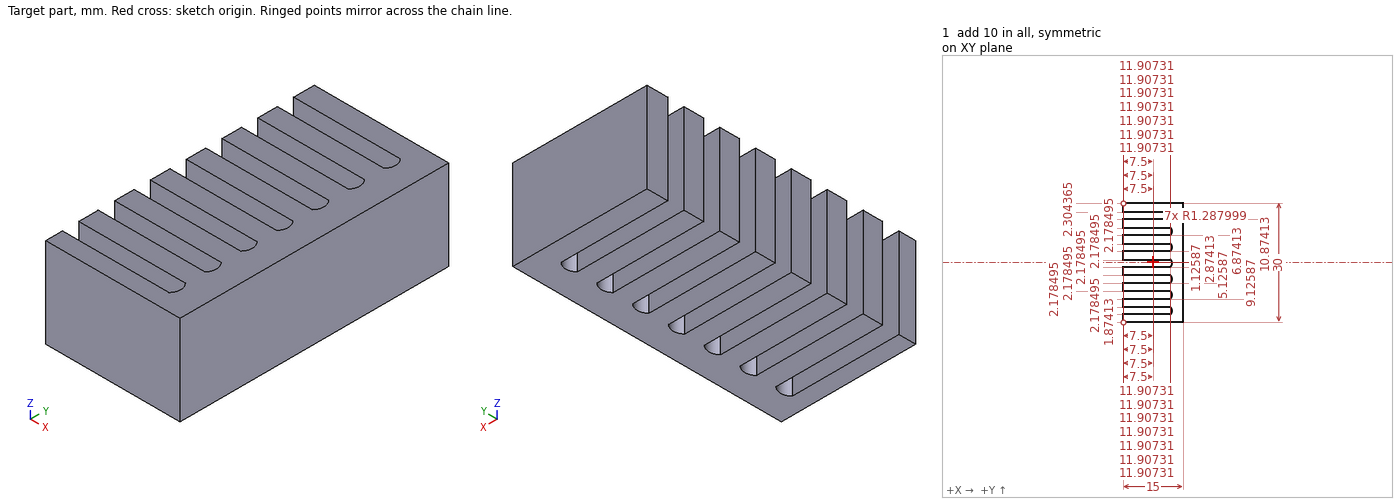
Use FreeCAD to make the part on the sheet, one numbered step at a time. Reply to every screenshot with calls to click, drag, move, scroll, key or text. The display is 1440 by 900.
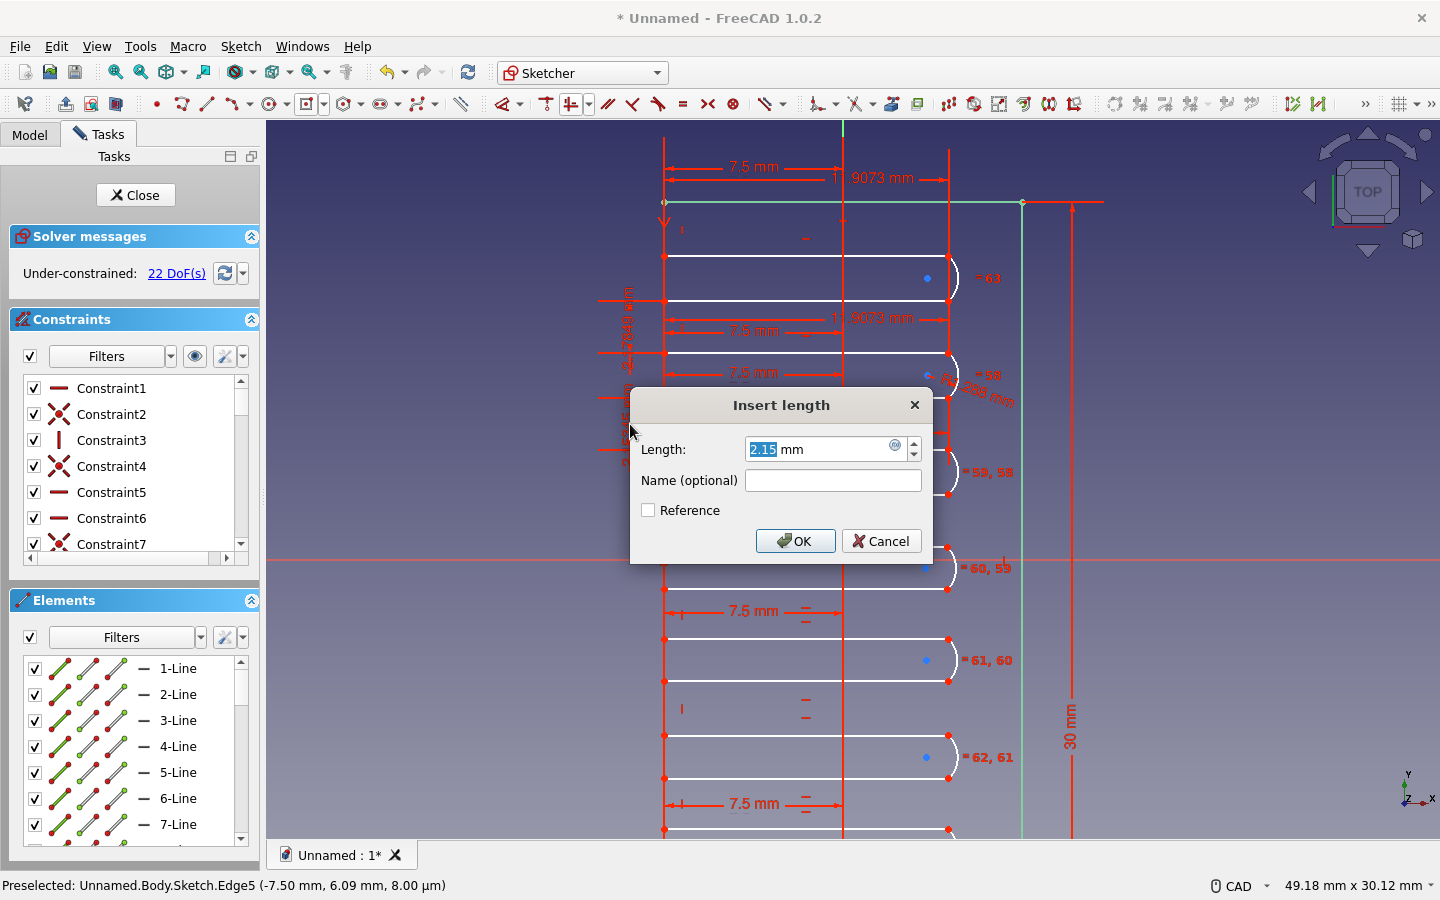
text(2.178495)
key(Return)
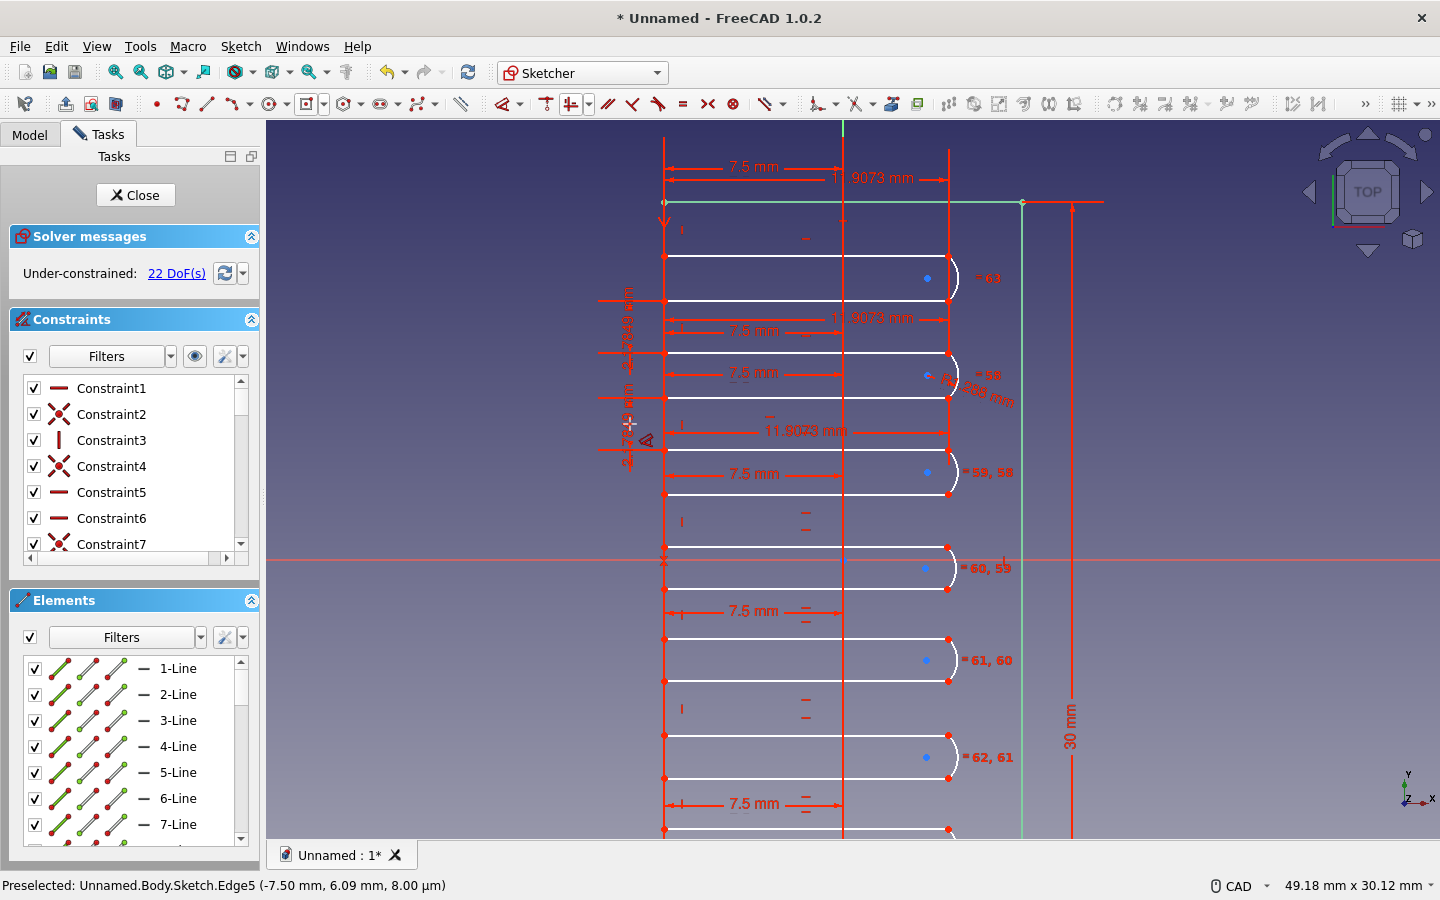
click(750, 450)
click(707, 416)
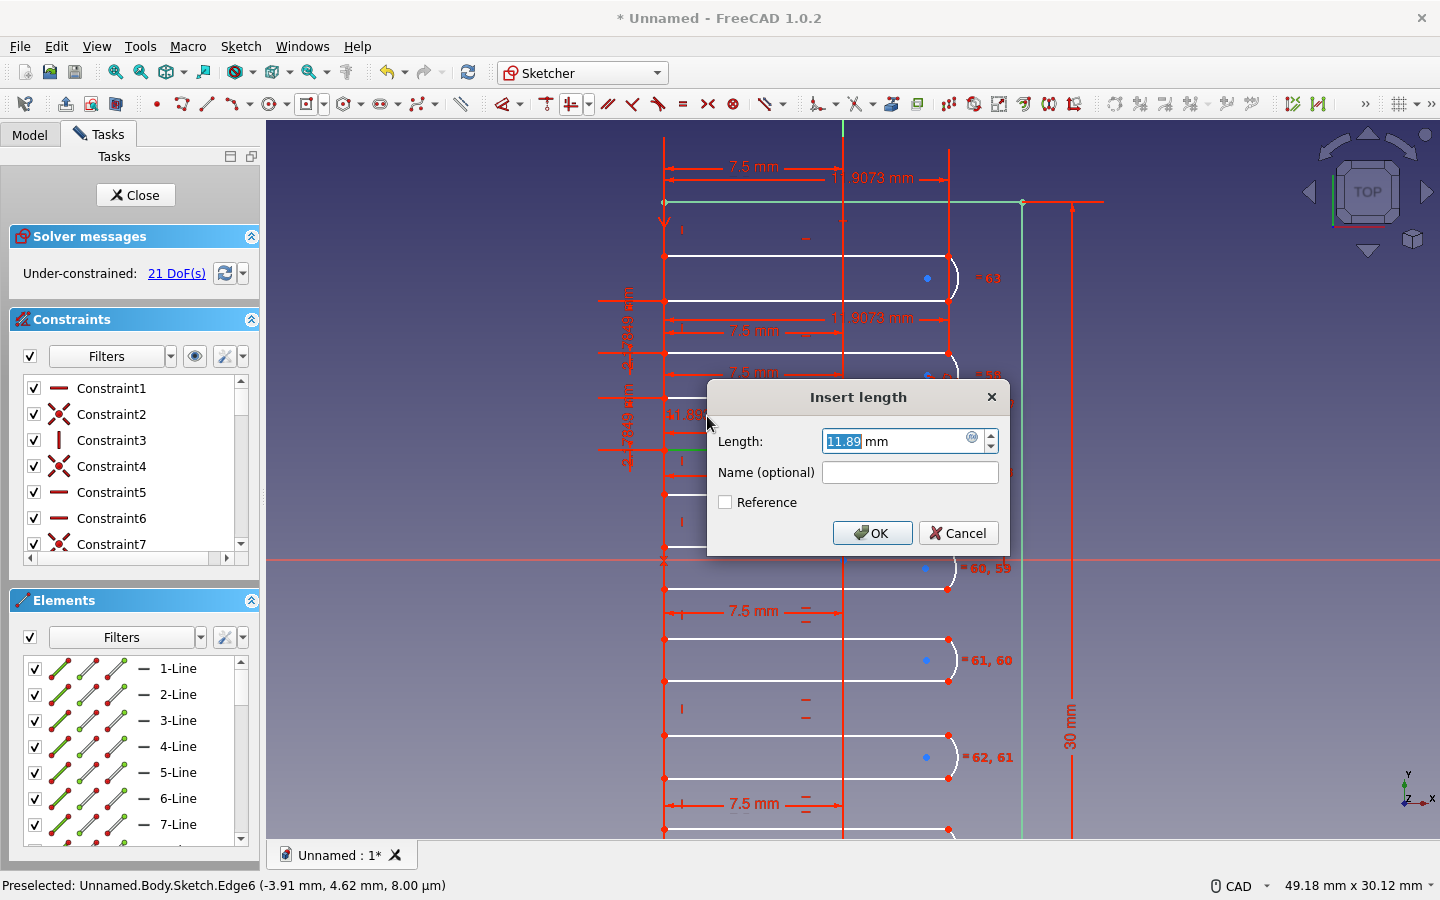
text(11.90731)
key(Return)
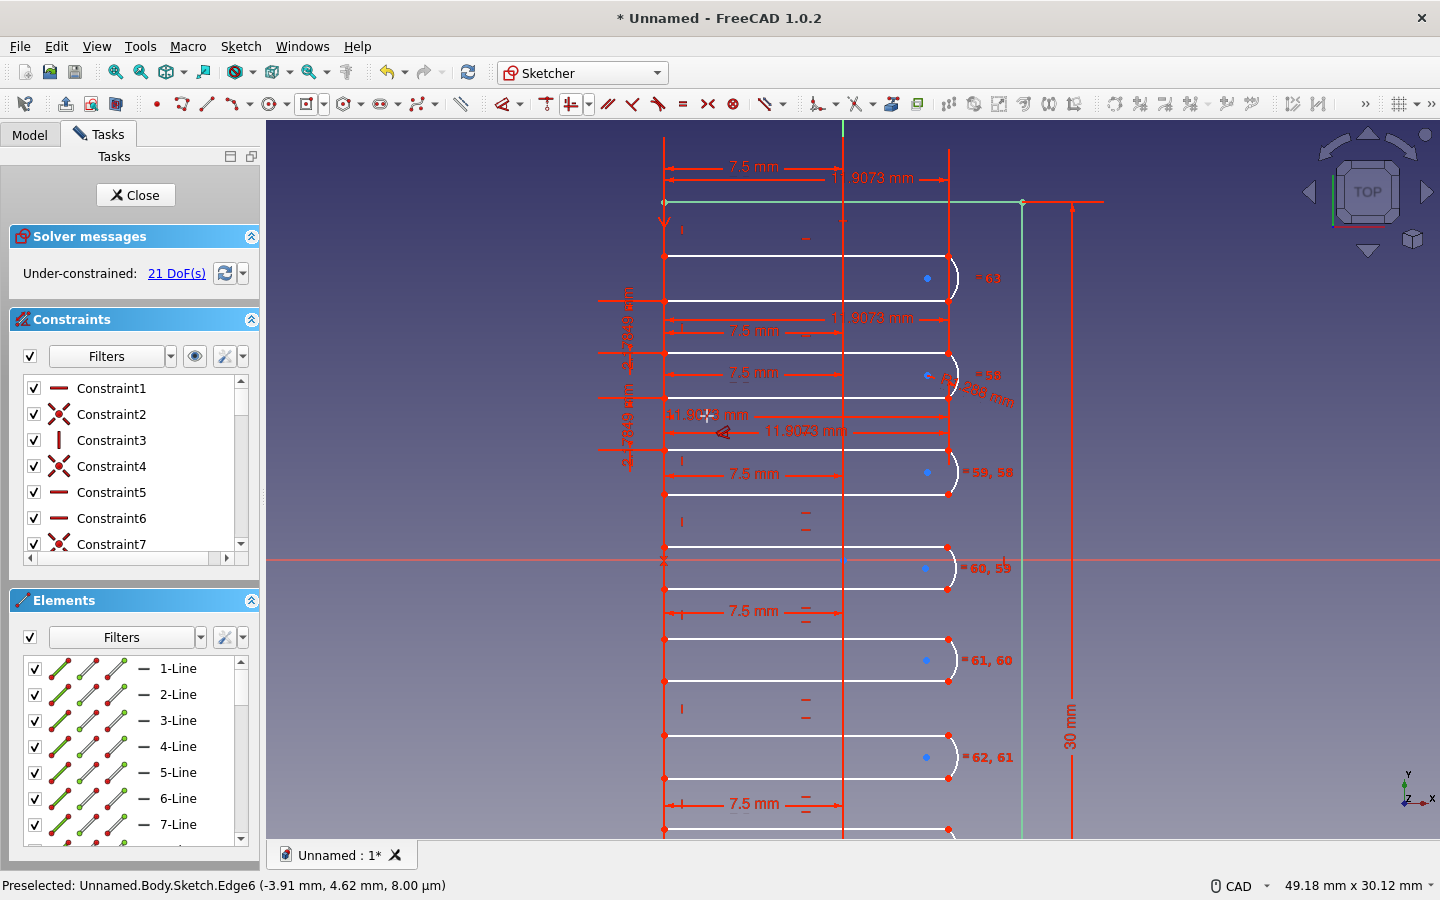
click(863, 495)
click(806, 529)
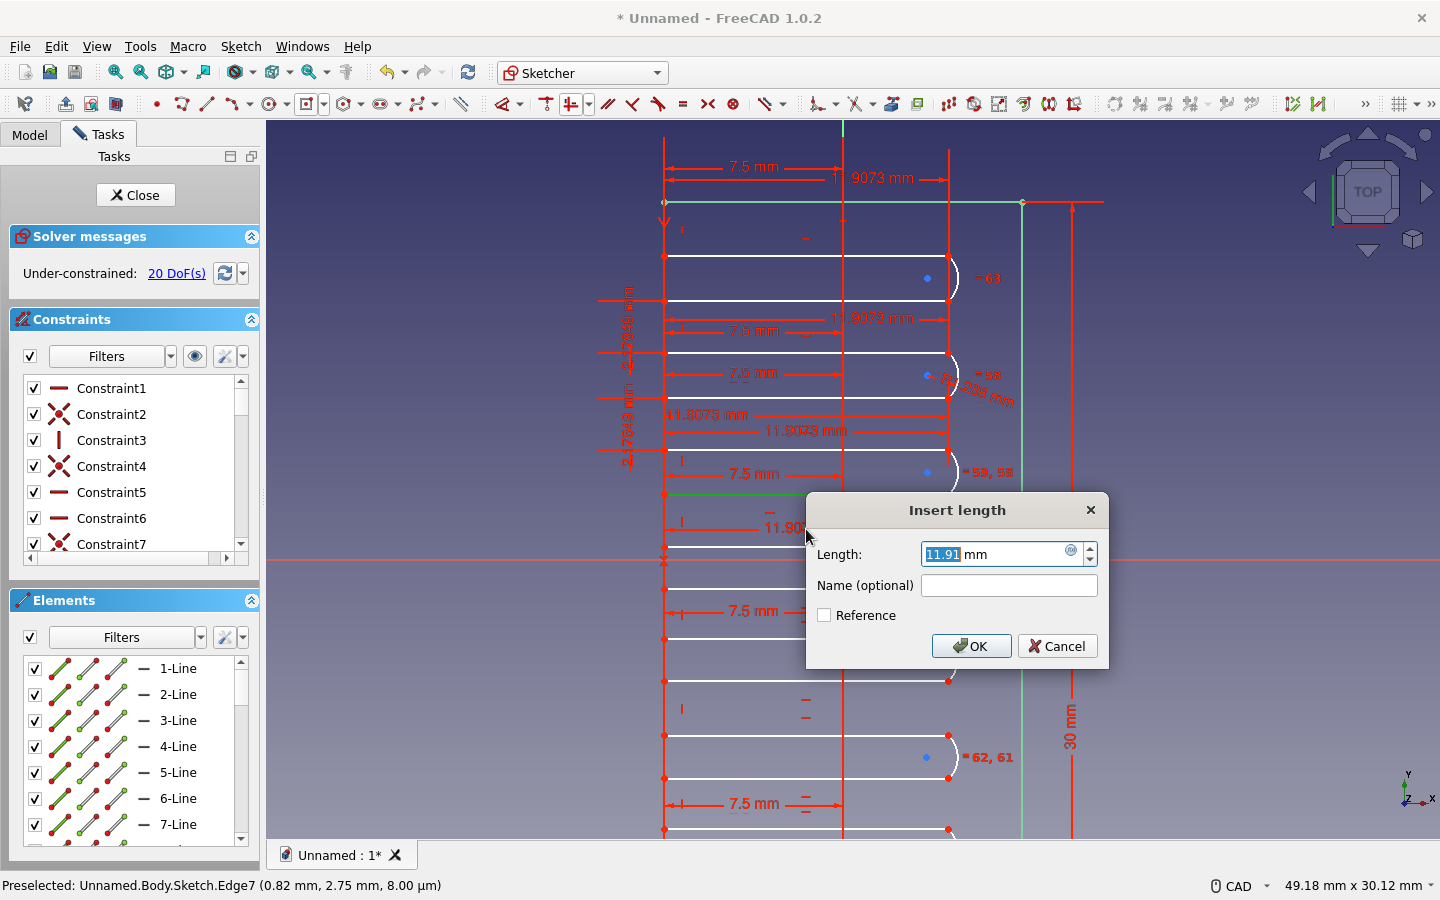
text(11.90731)
key(Return)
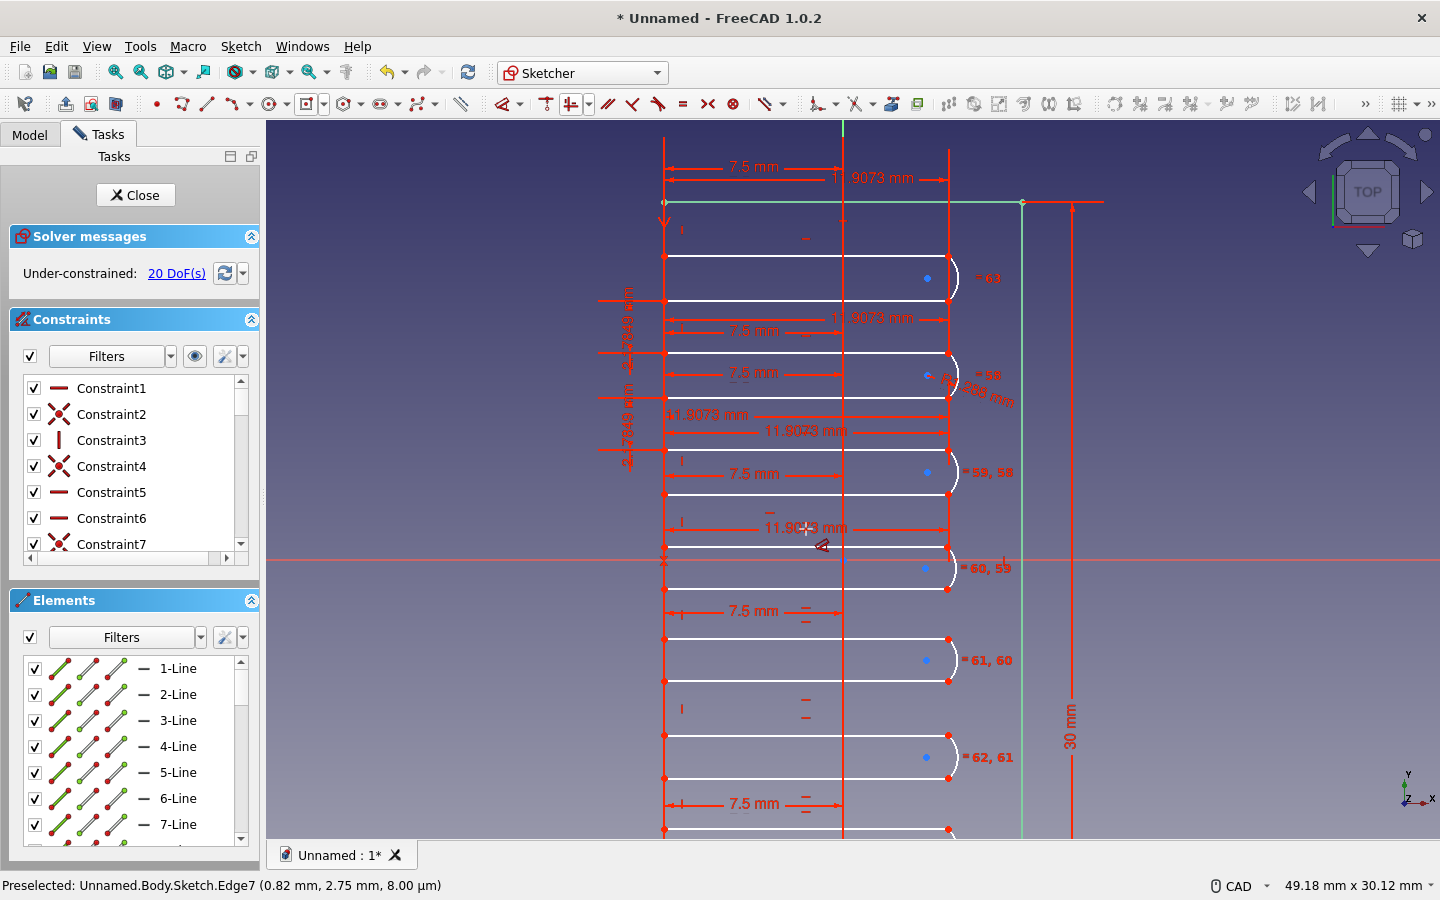
click(664, 511)
click(630, 521)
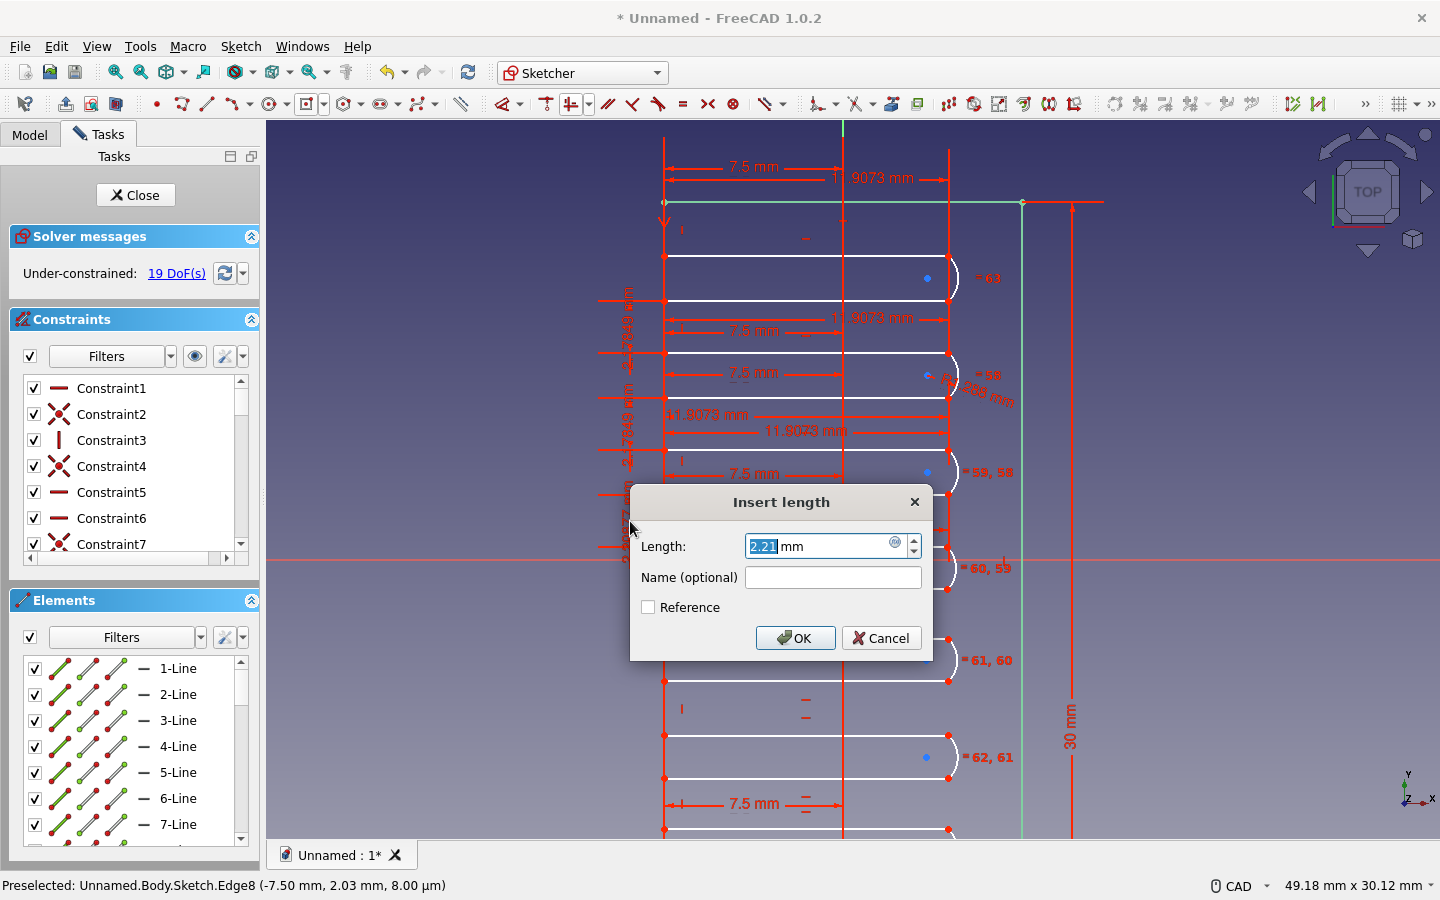
text(2.178495)
key(Return)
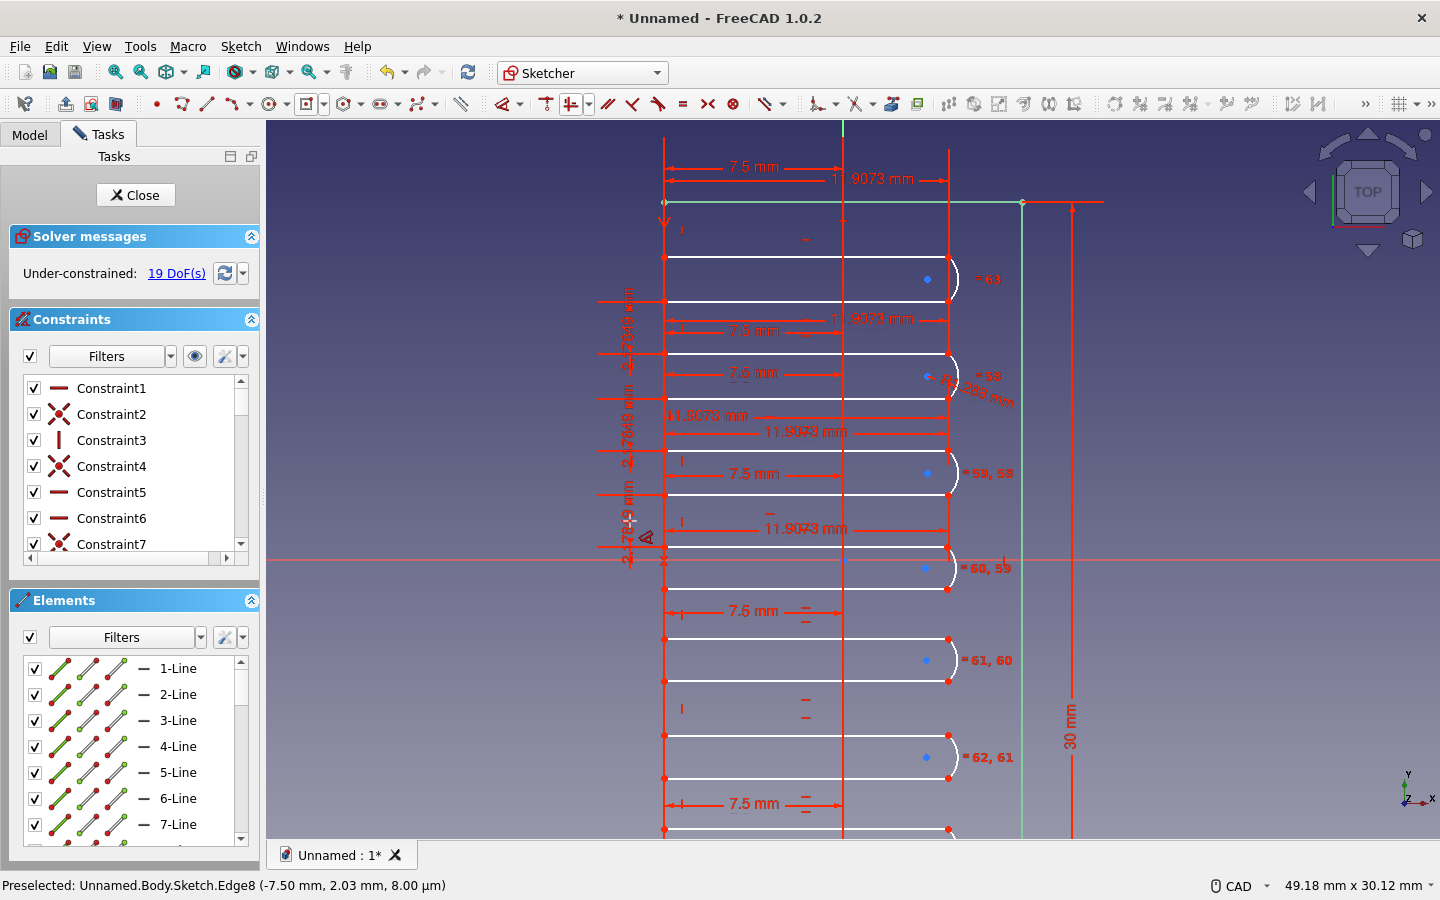
click(749, 547)
click(707, 513)